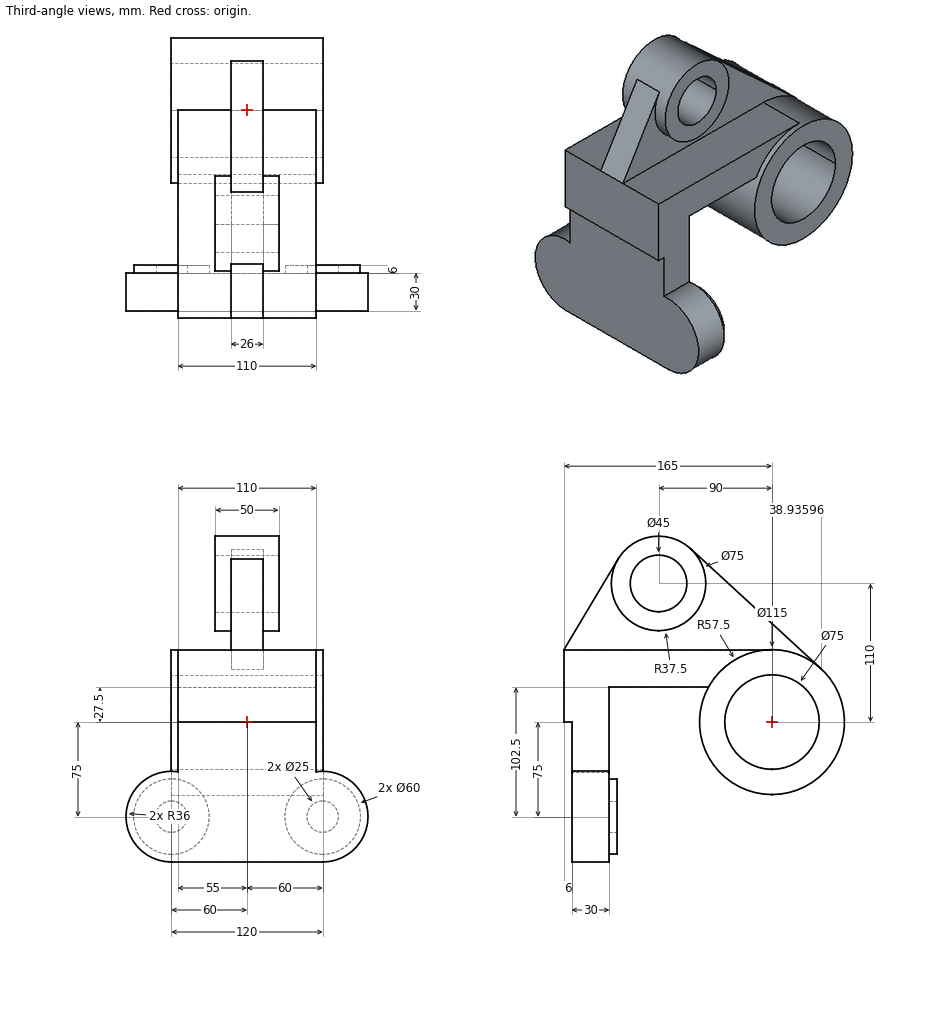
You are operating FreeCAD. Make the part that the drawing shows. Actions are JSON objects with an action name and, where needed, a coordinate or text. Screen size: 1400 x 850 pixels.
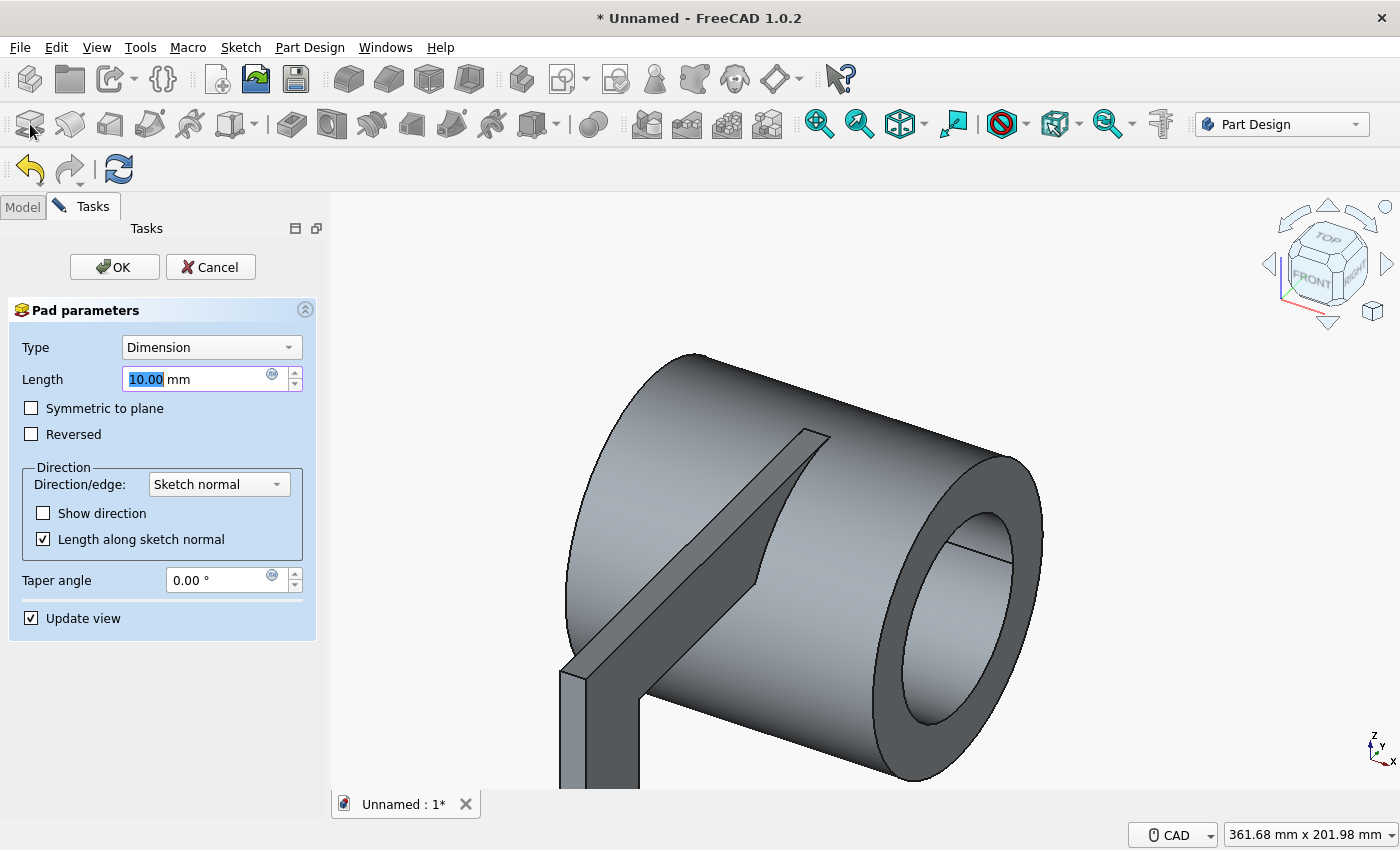
{"action": "type", "text": "110"}
{"action": "key", "text": "Tab"}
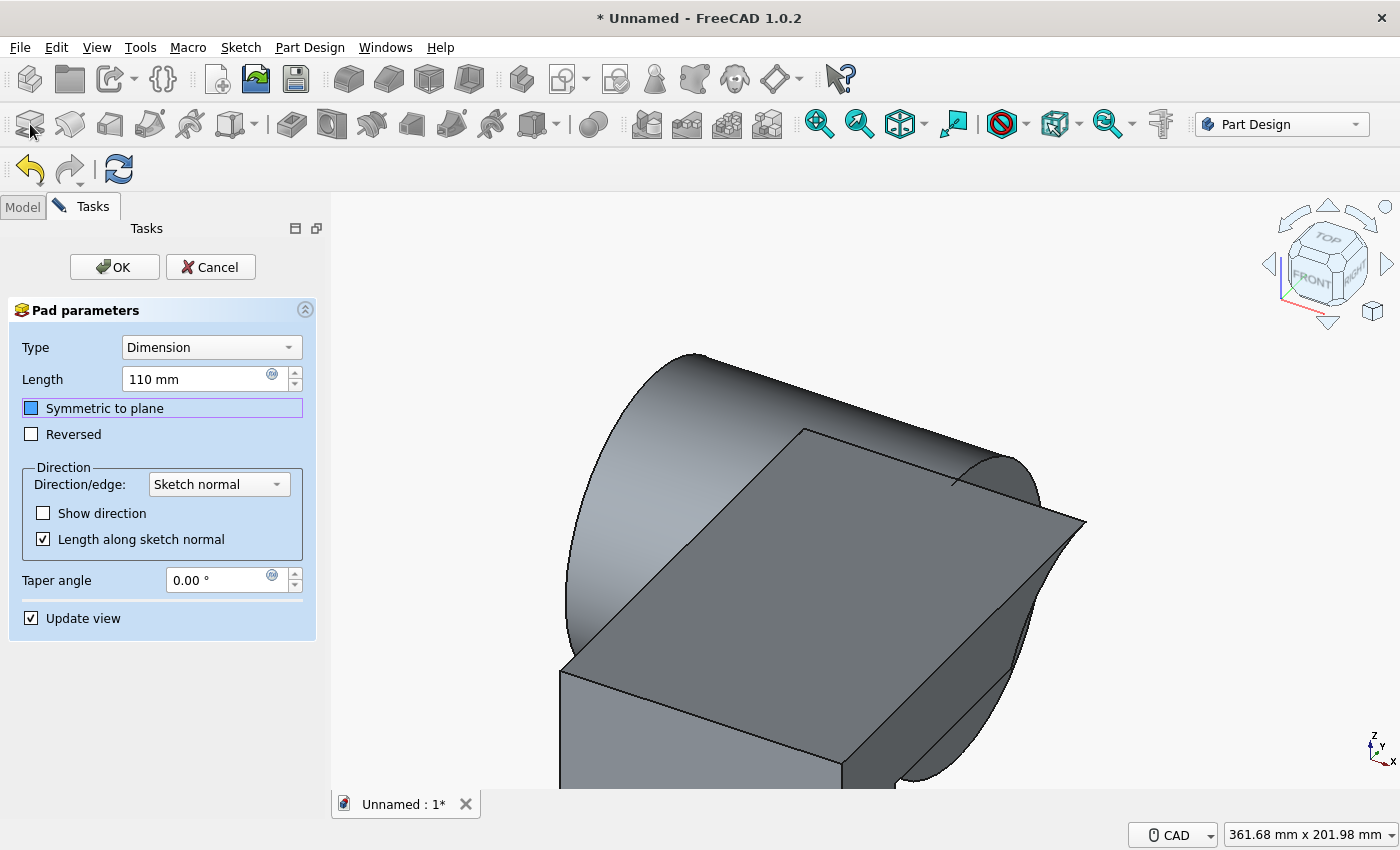
{"action": "left_click", "coordinate": [30, 408]}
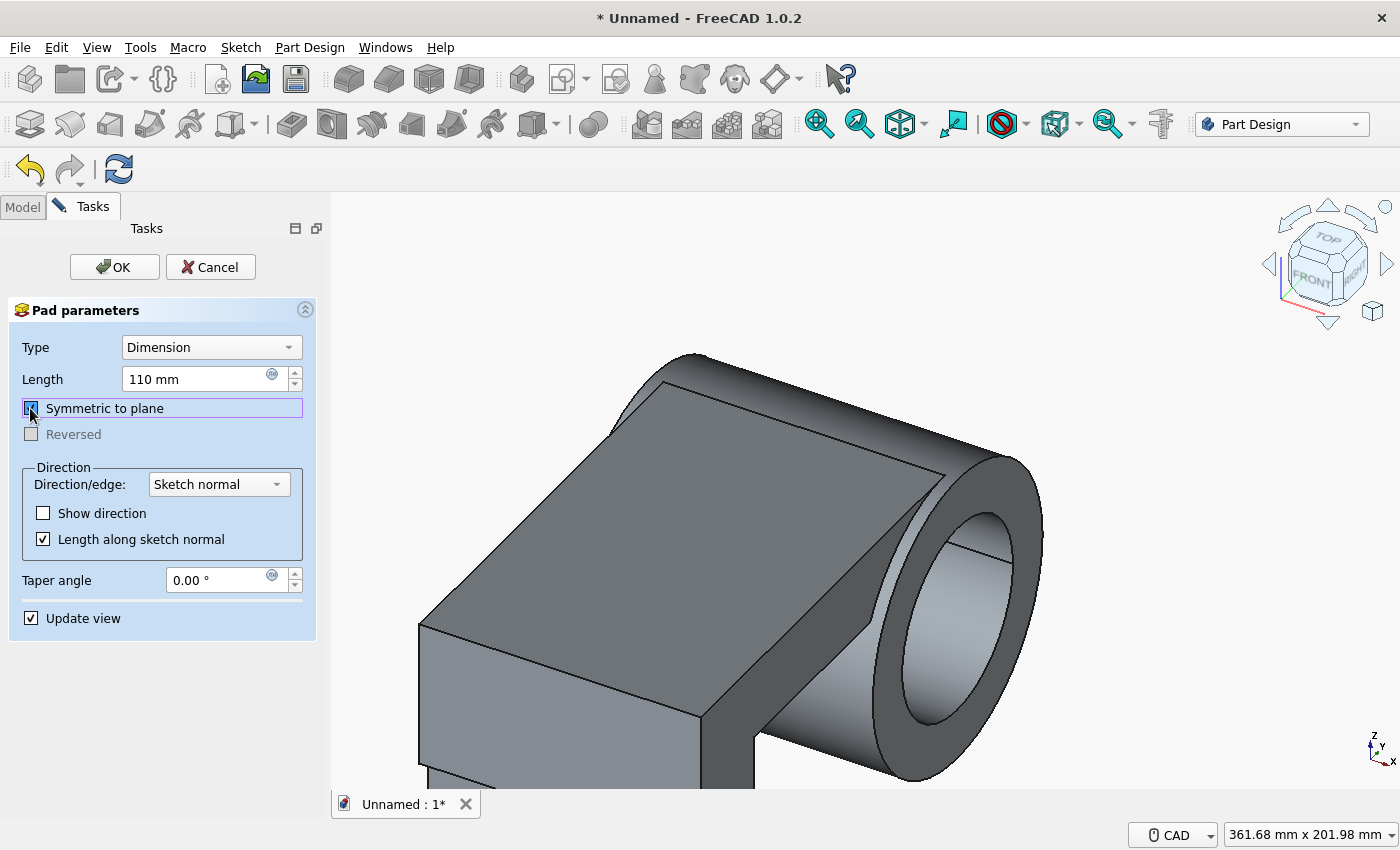
{"action": "left_click", "coordinate": [115, 267]}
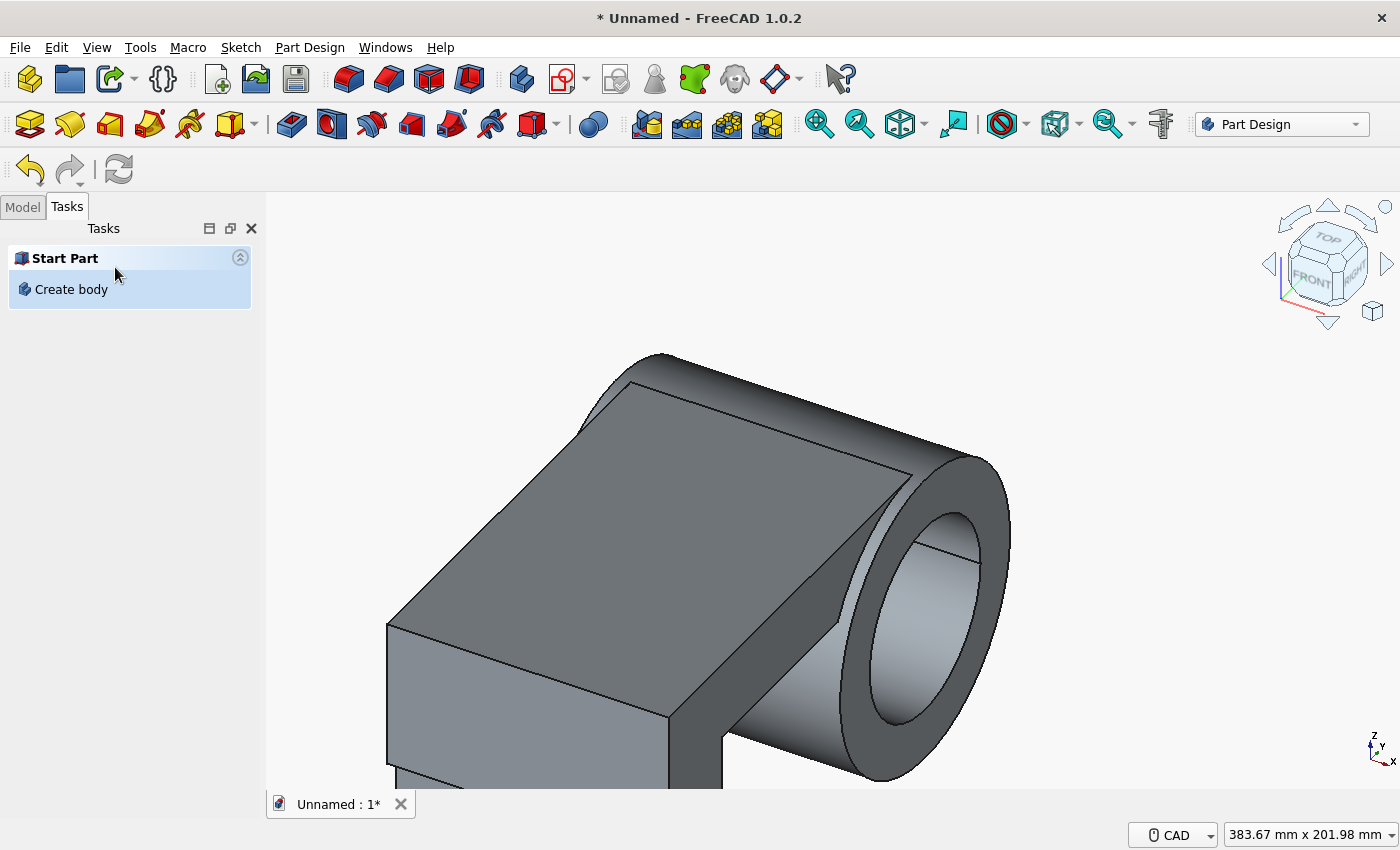
{"action": "left_click", "coordinate": [820, 124]}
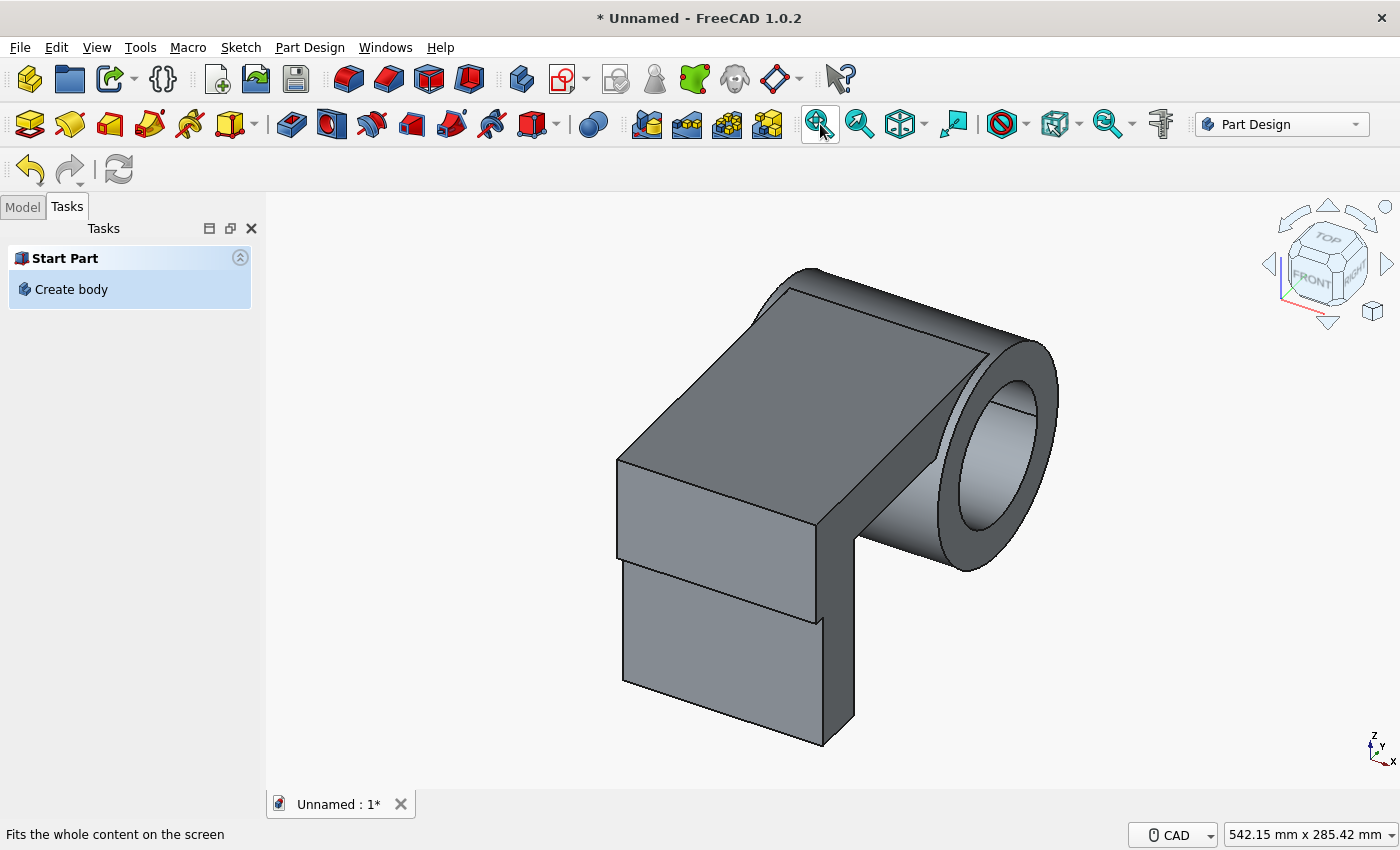
{"action": "left_click", "coordinate": [522, 80]}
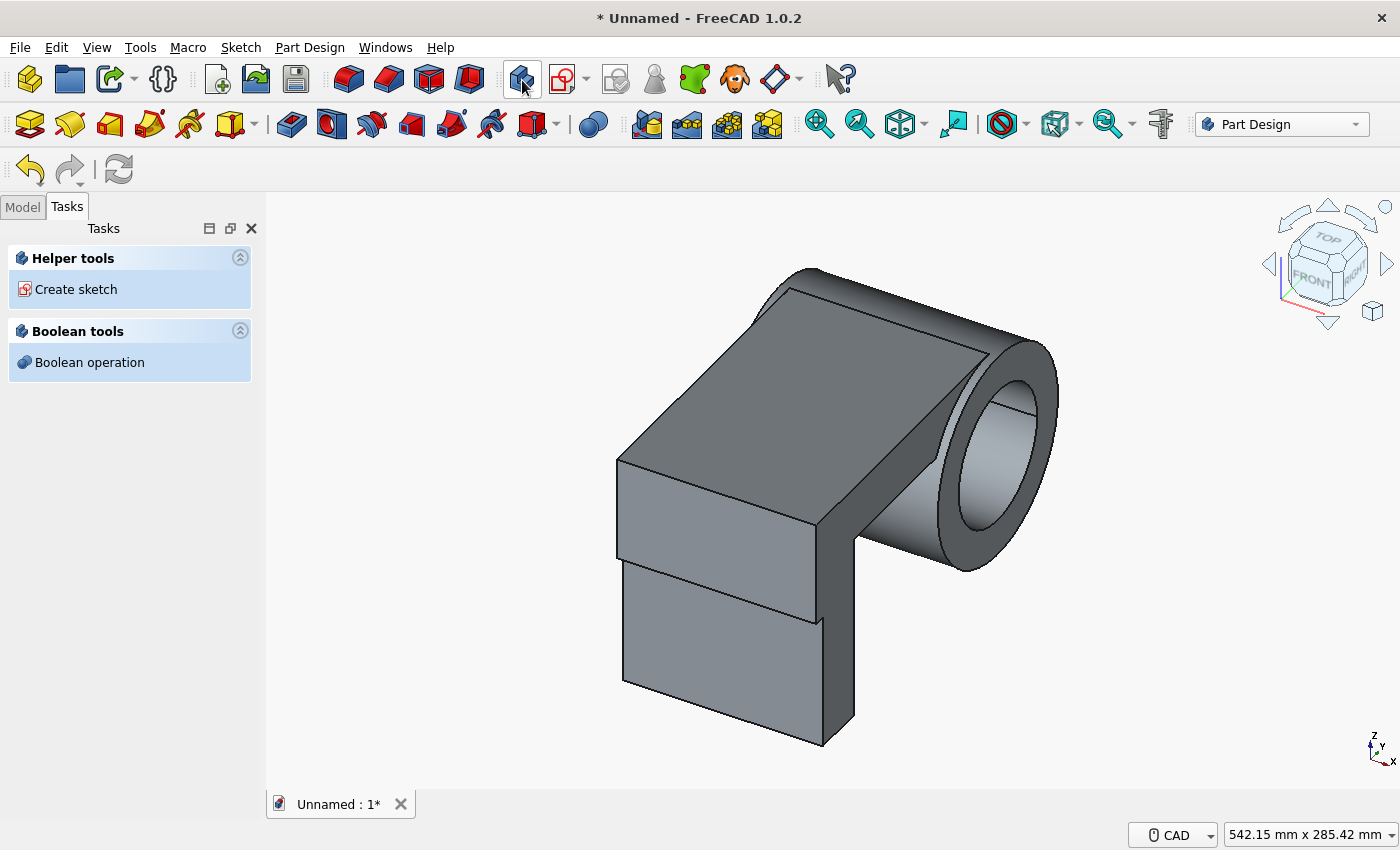
{"action": "left_click", "coordinate": [306, 749]}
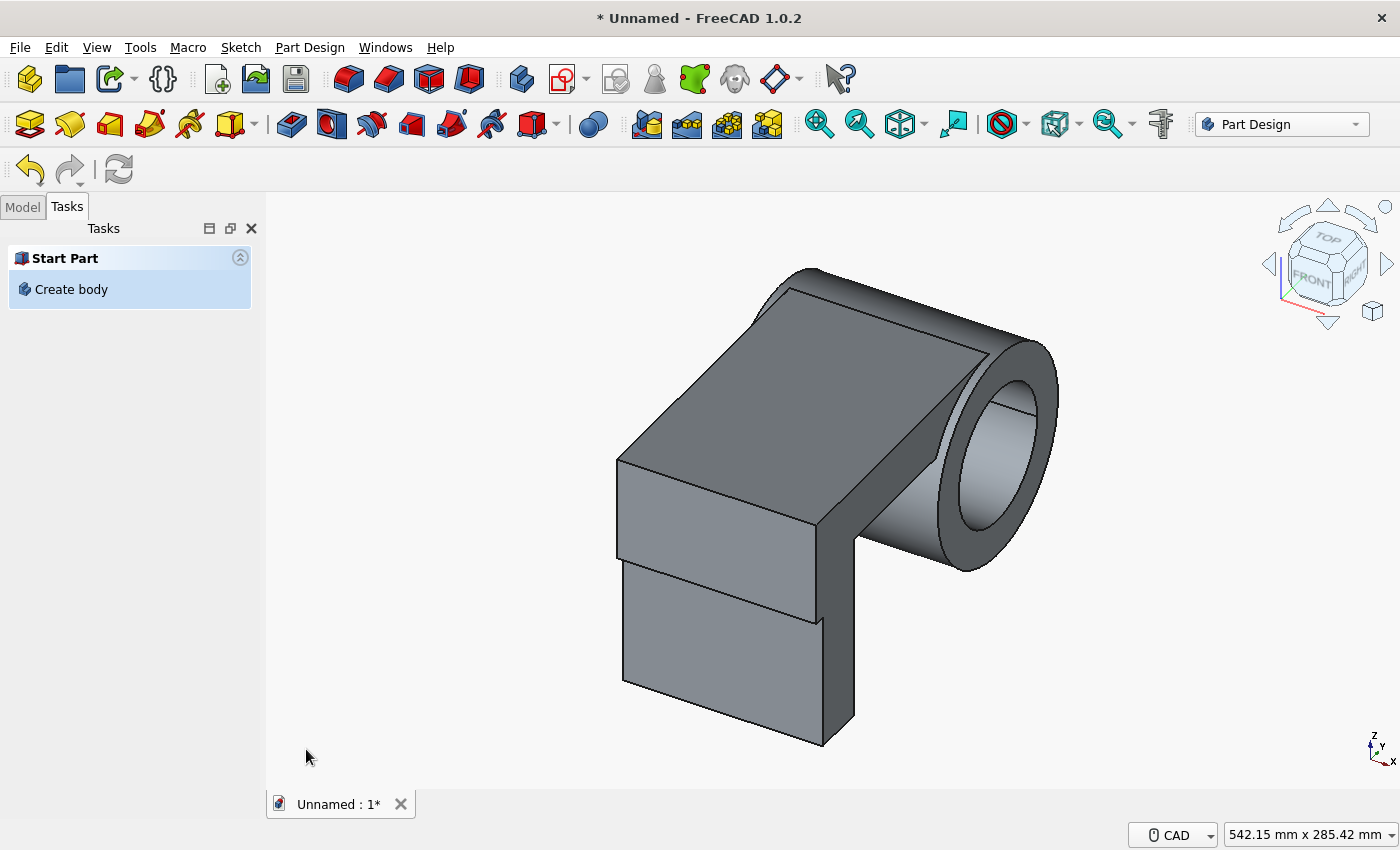
{"action": "left_click", "coordinate": [562, 80]}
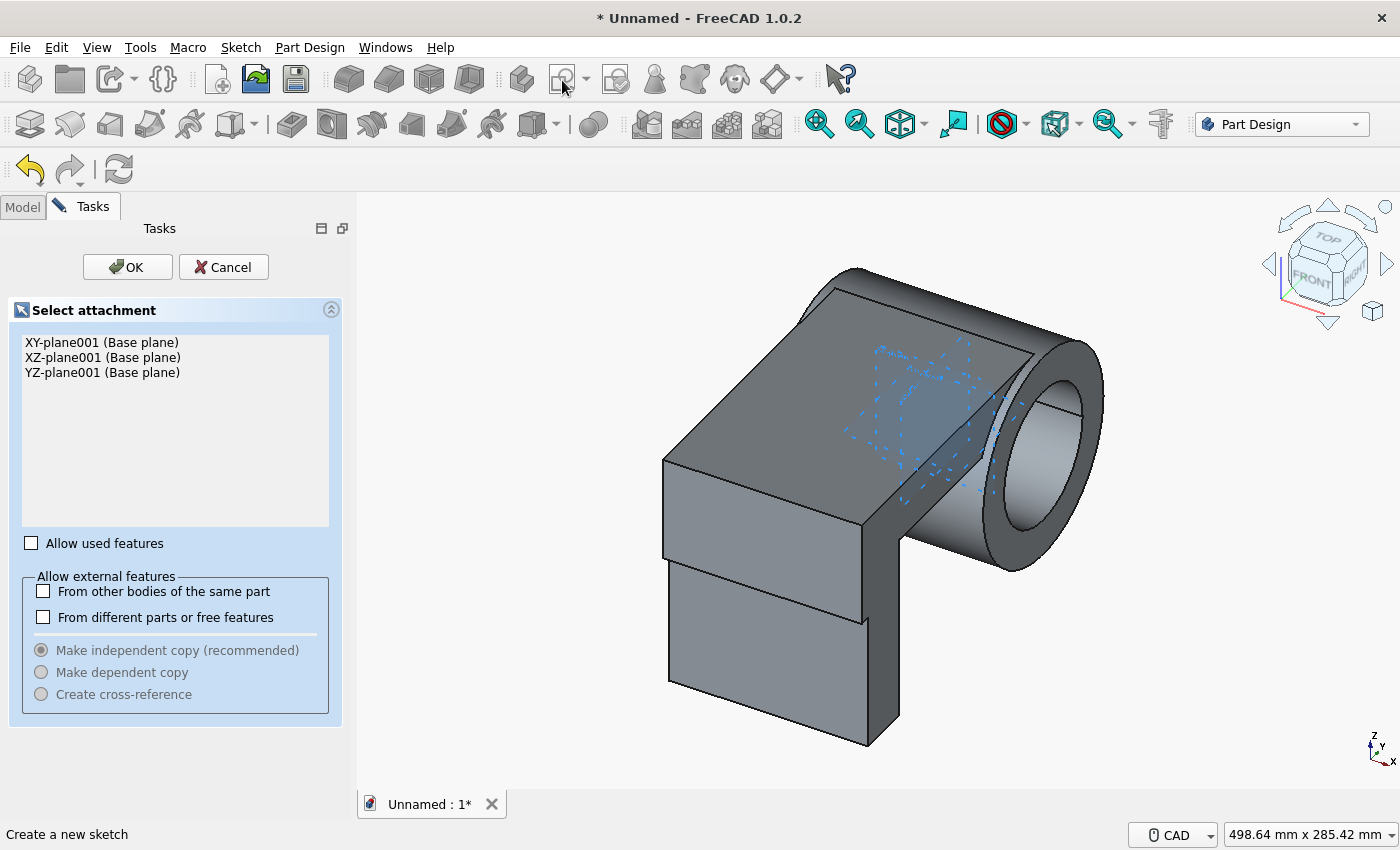
{"action": "left_click", "coordinate": [82, 372]}